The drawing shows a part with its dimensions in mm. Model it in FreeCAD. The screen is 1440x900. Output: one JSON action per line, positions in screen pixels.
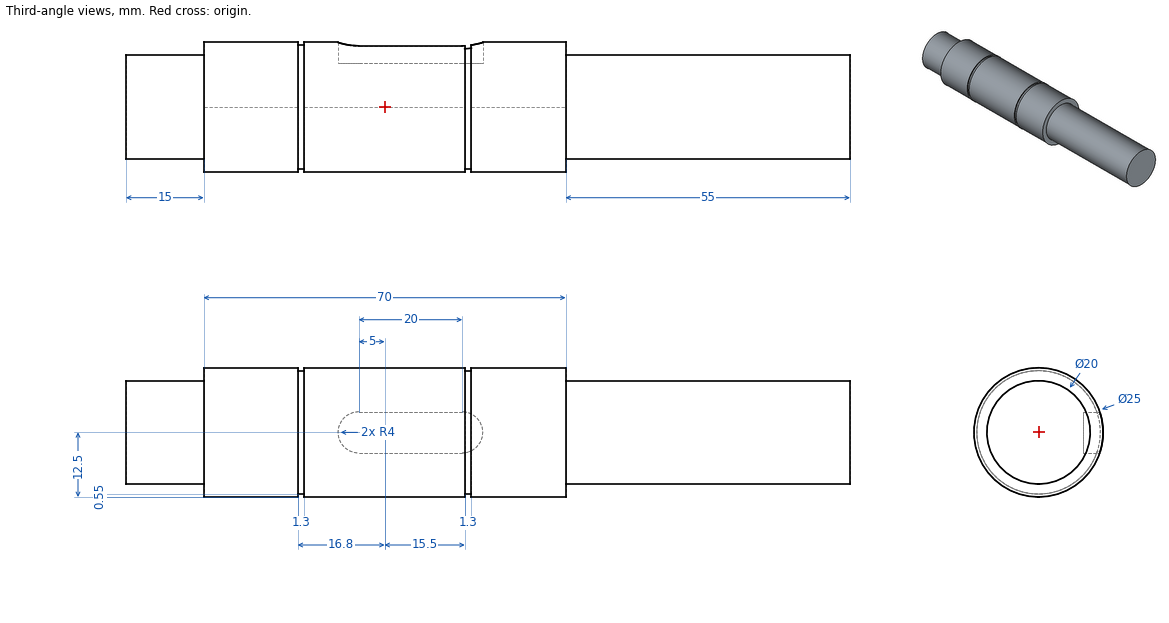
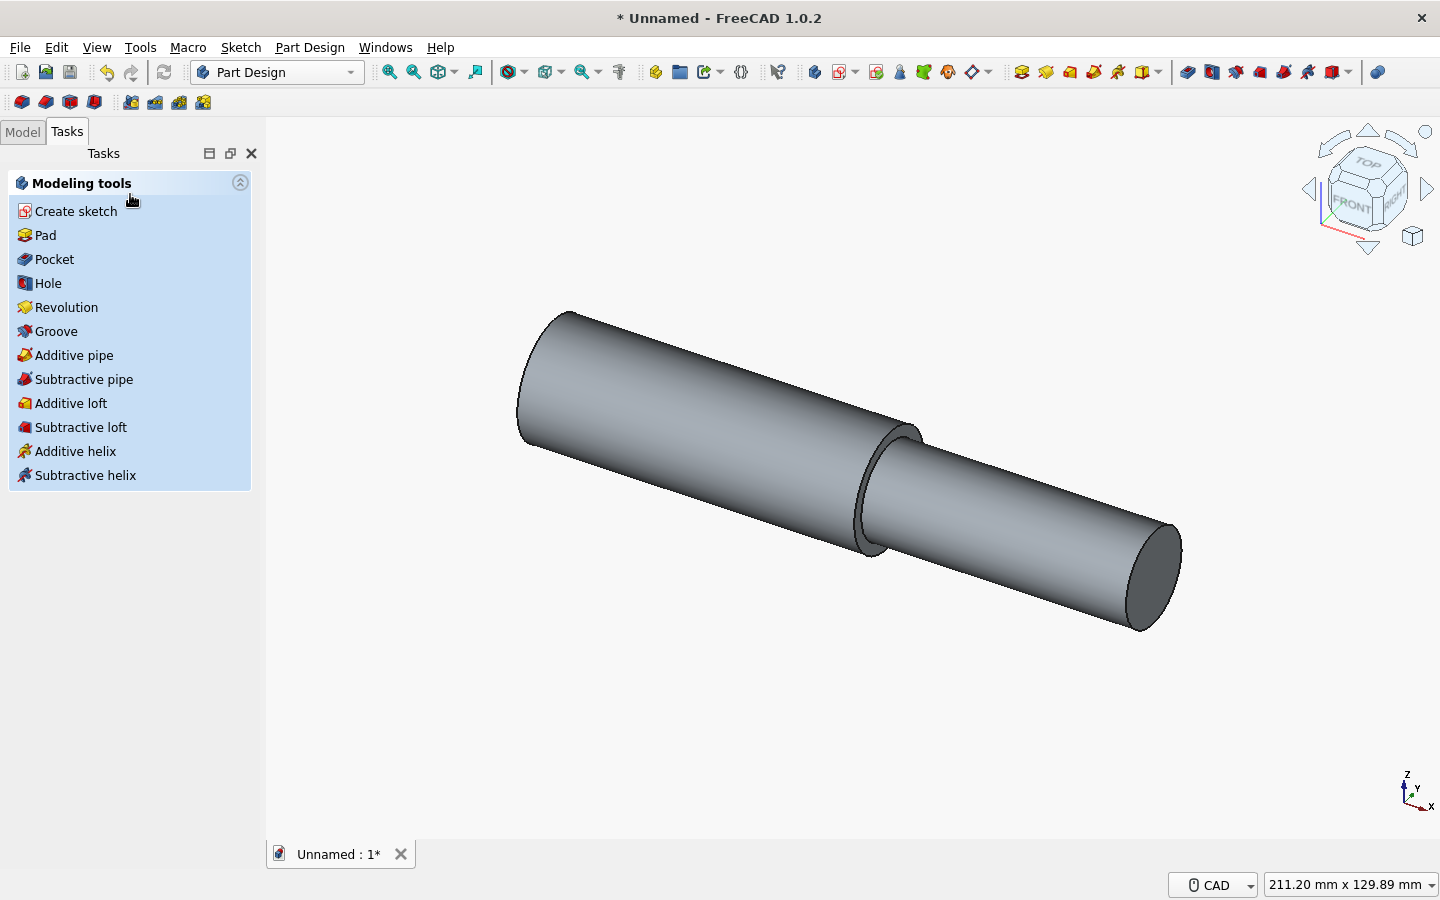
{"action": "left_click", "coordinate": [1236, 72]}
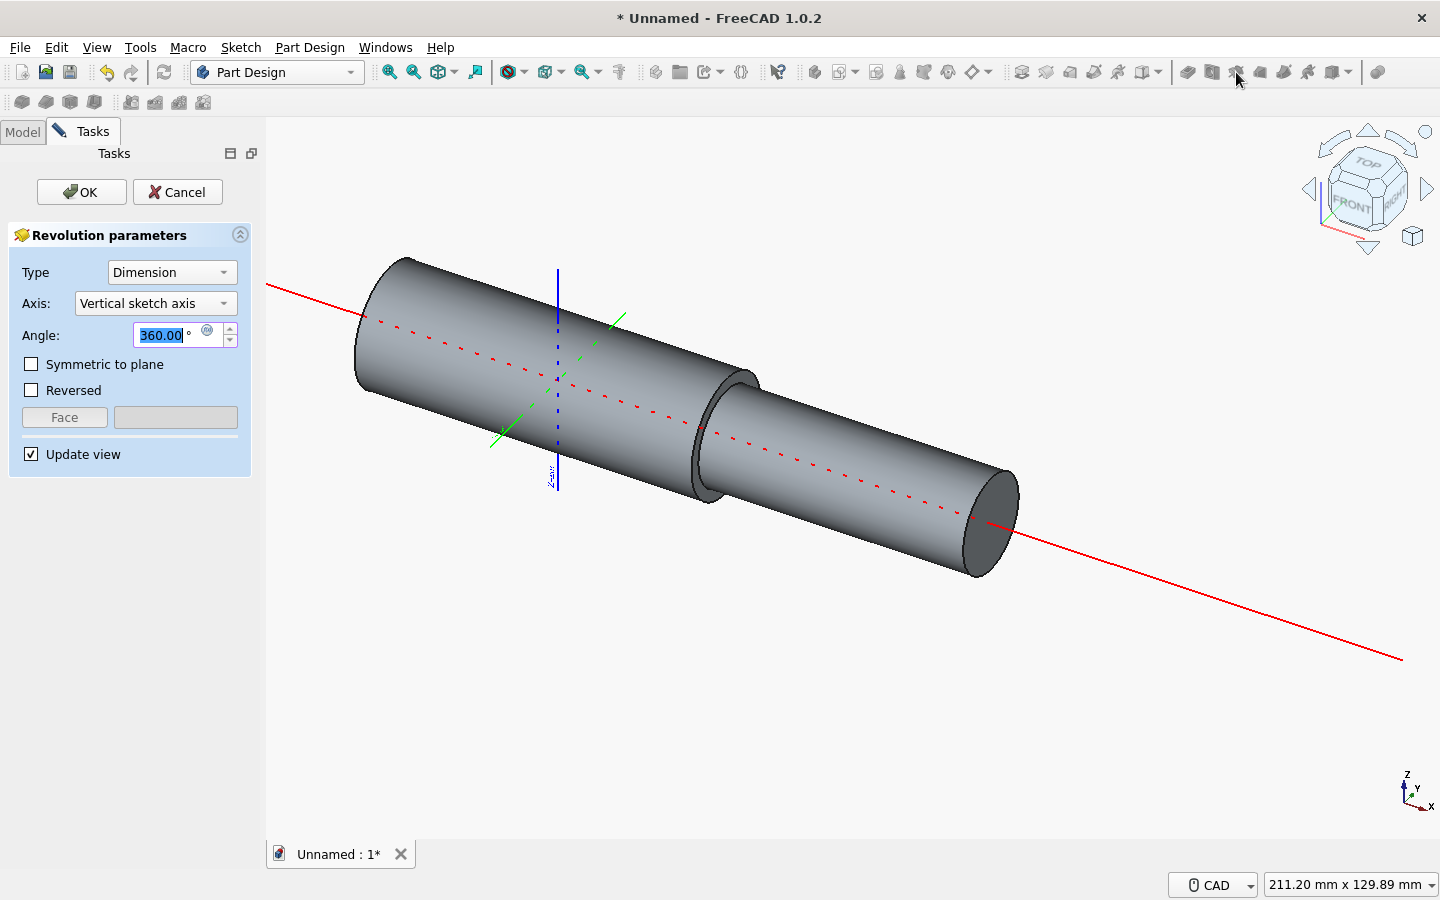
{"action": "left_click", "coordinate": [156, 304]}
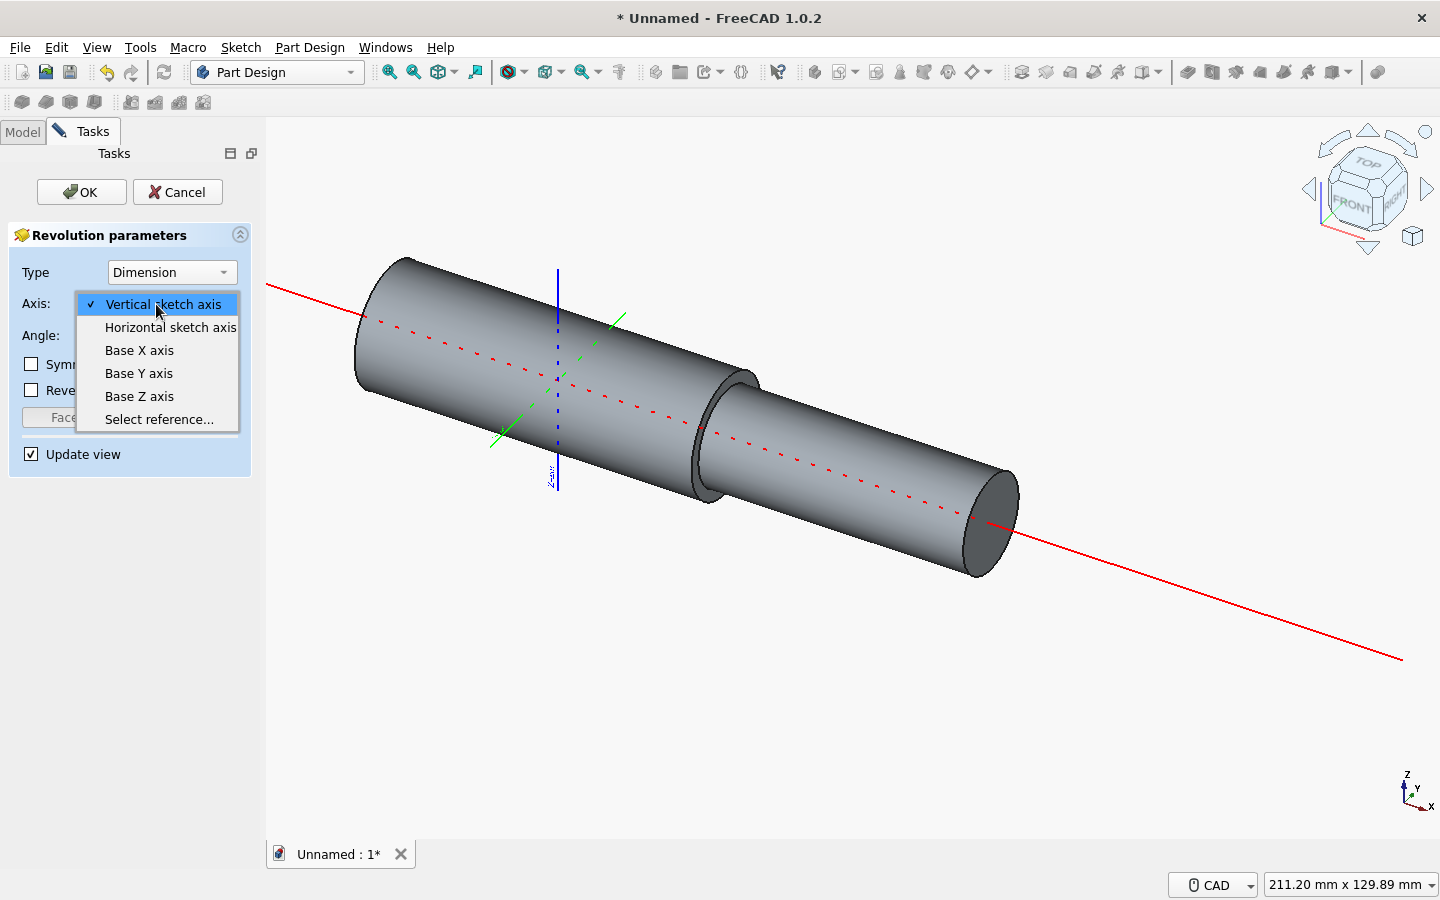
{"action": "left_click", "coordinate": [156, 328]}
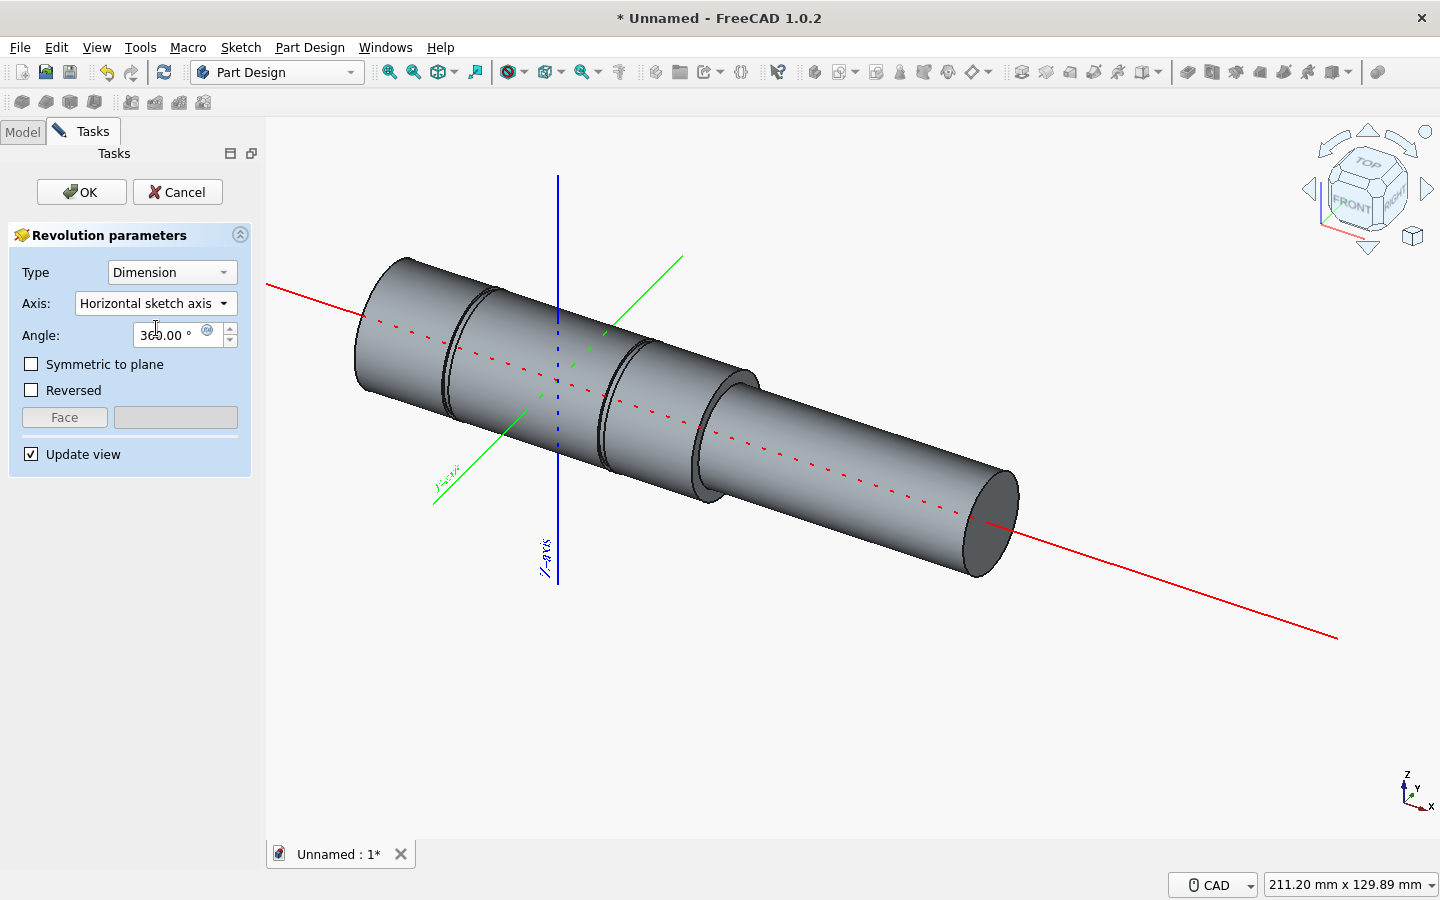
{"action": "left_click", "coordinate": [82, 192]}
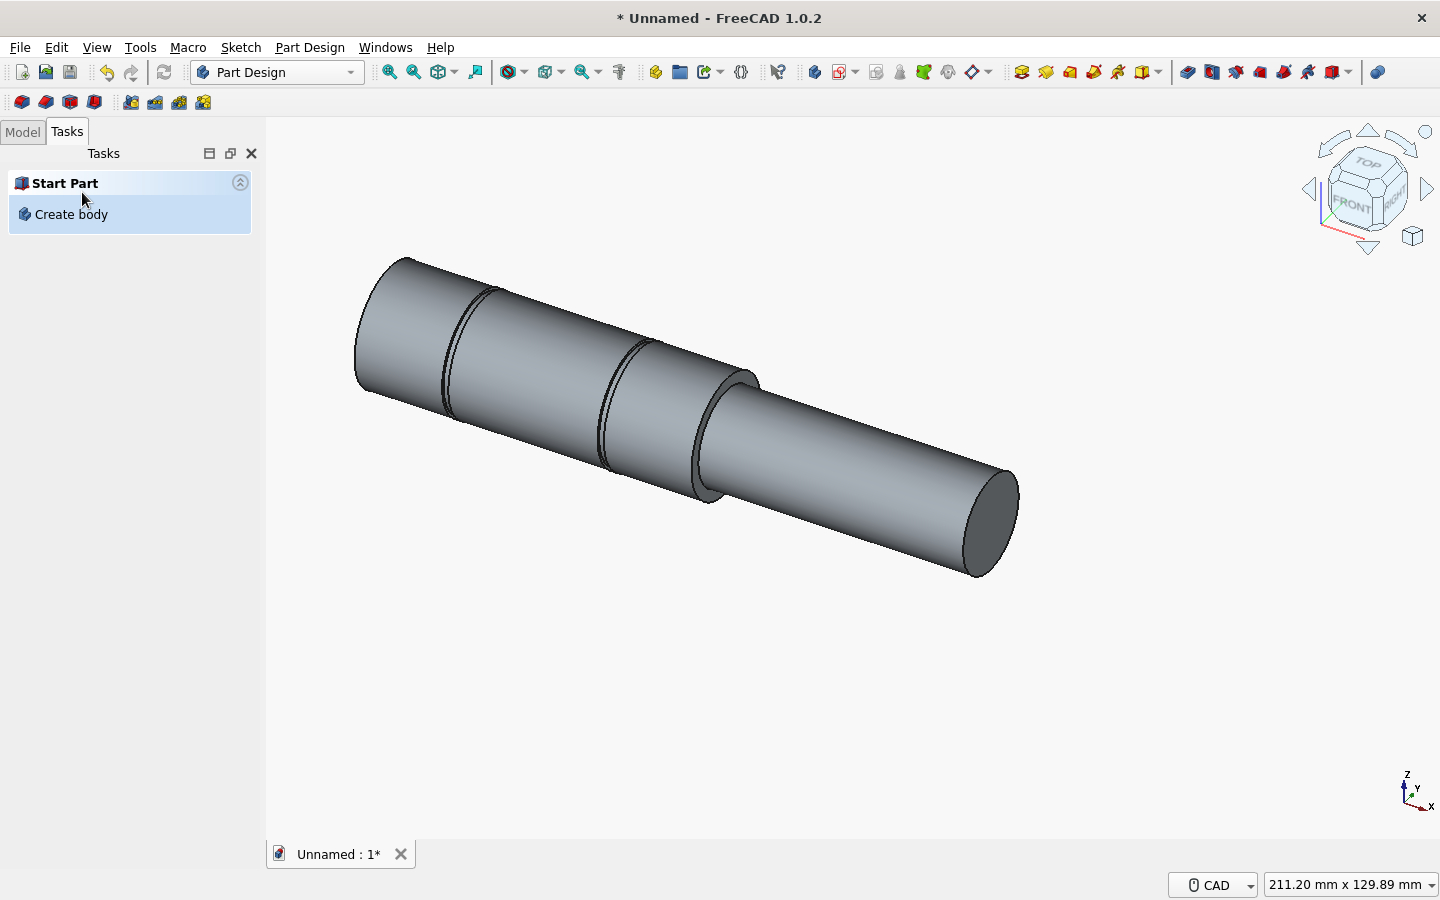
{"action": "left_click", "coordinate": [23, 131]}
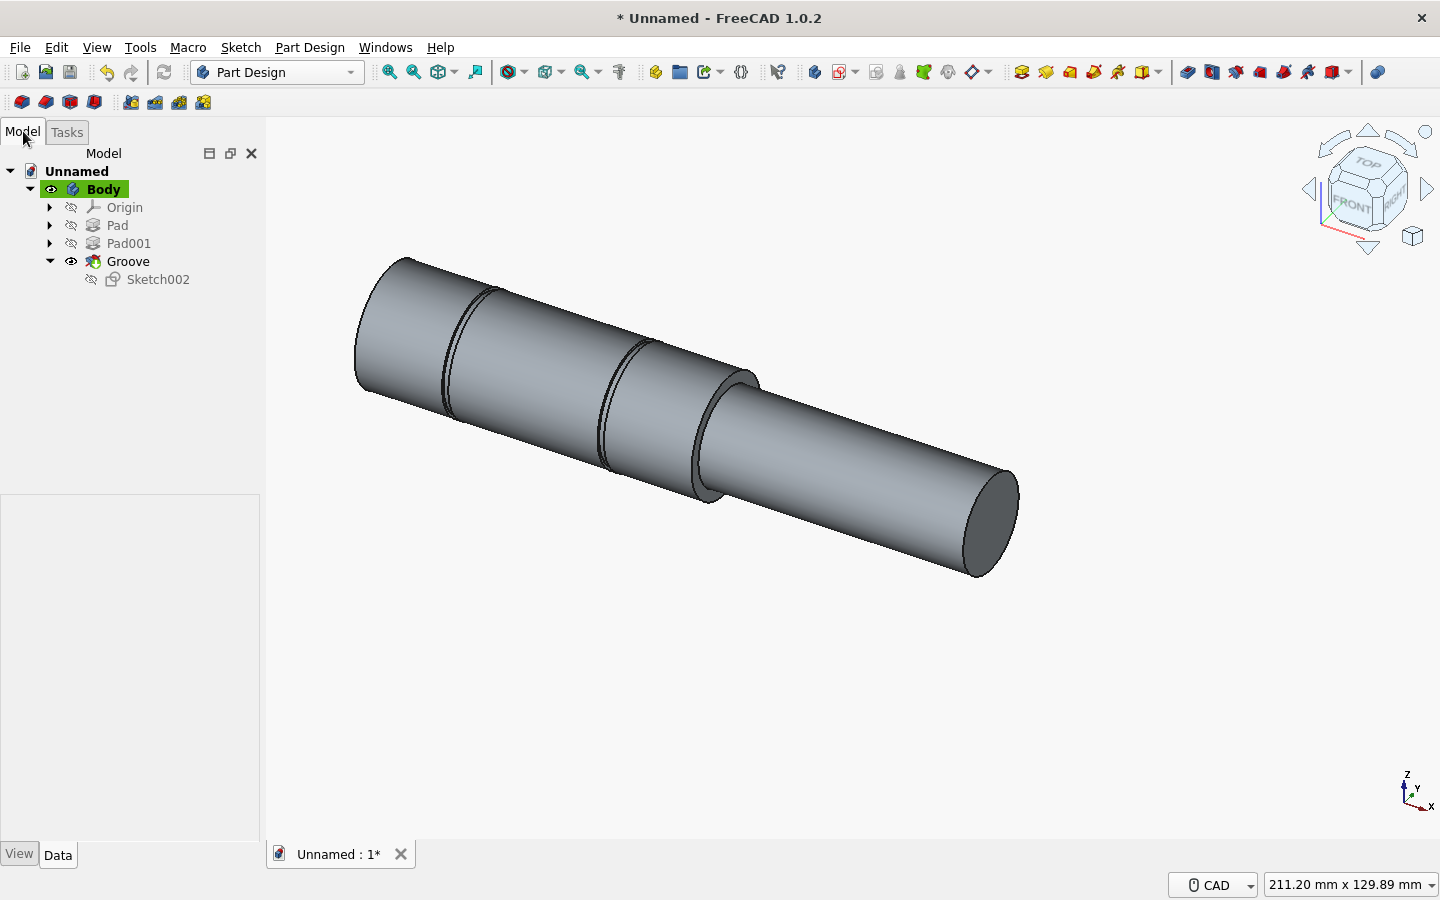
{"action": "left_click", "coordinate": [50, 207]}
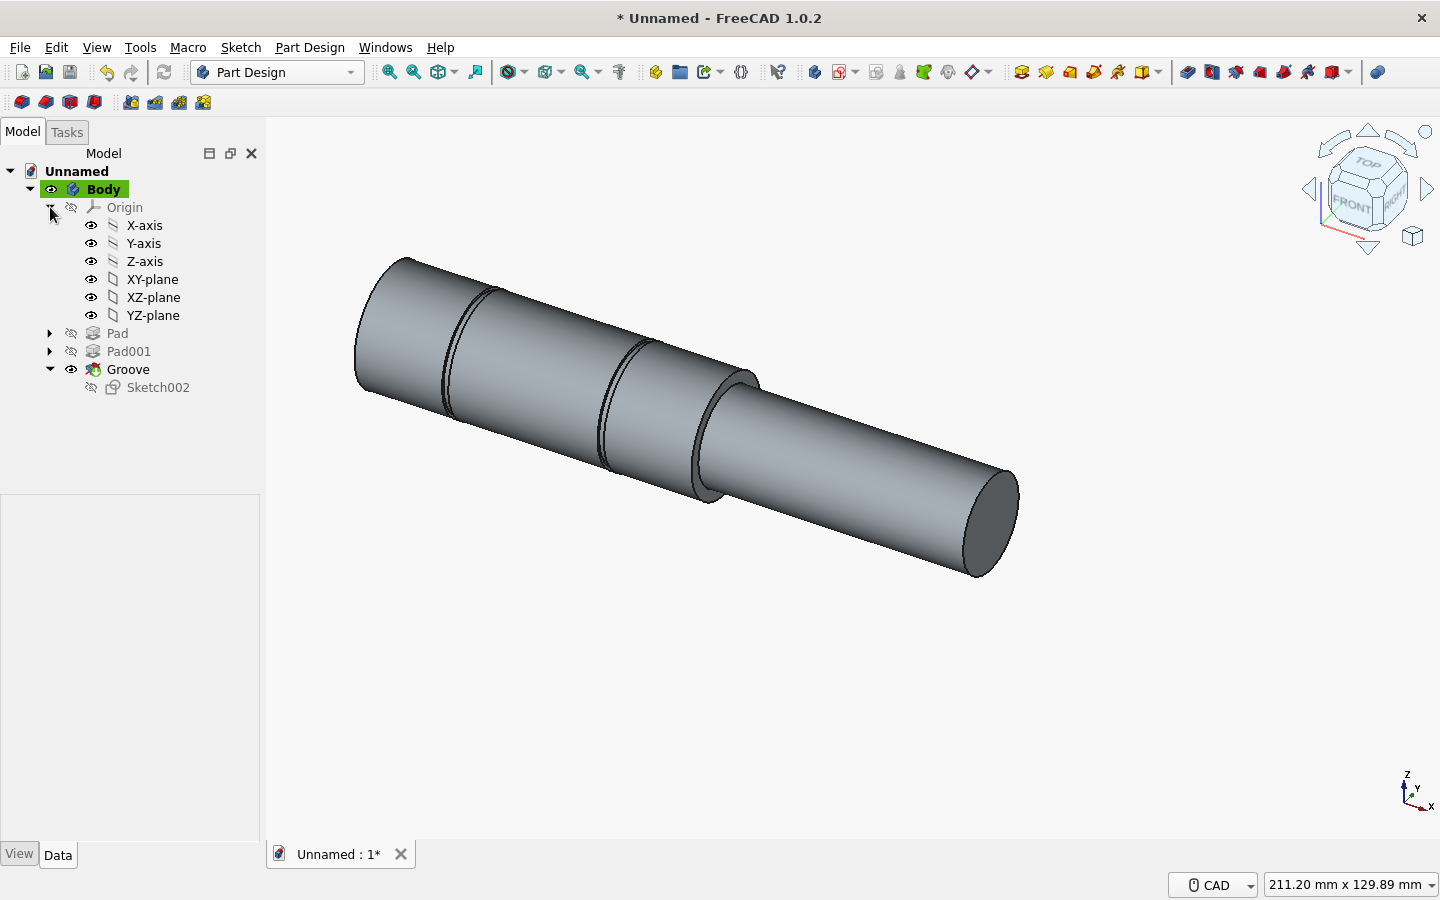
{"action": "left_click", "coordinate": [136, 297]}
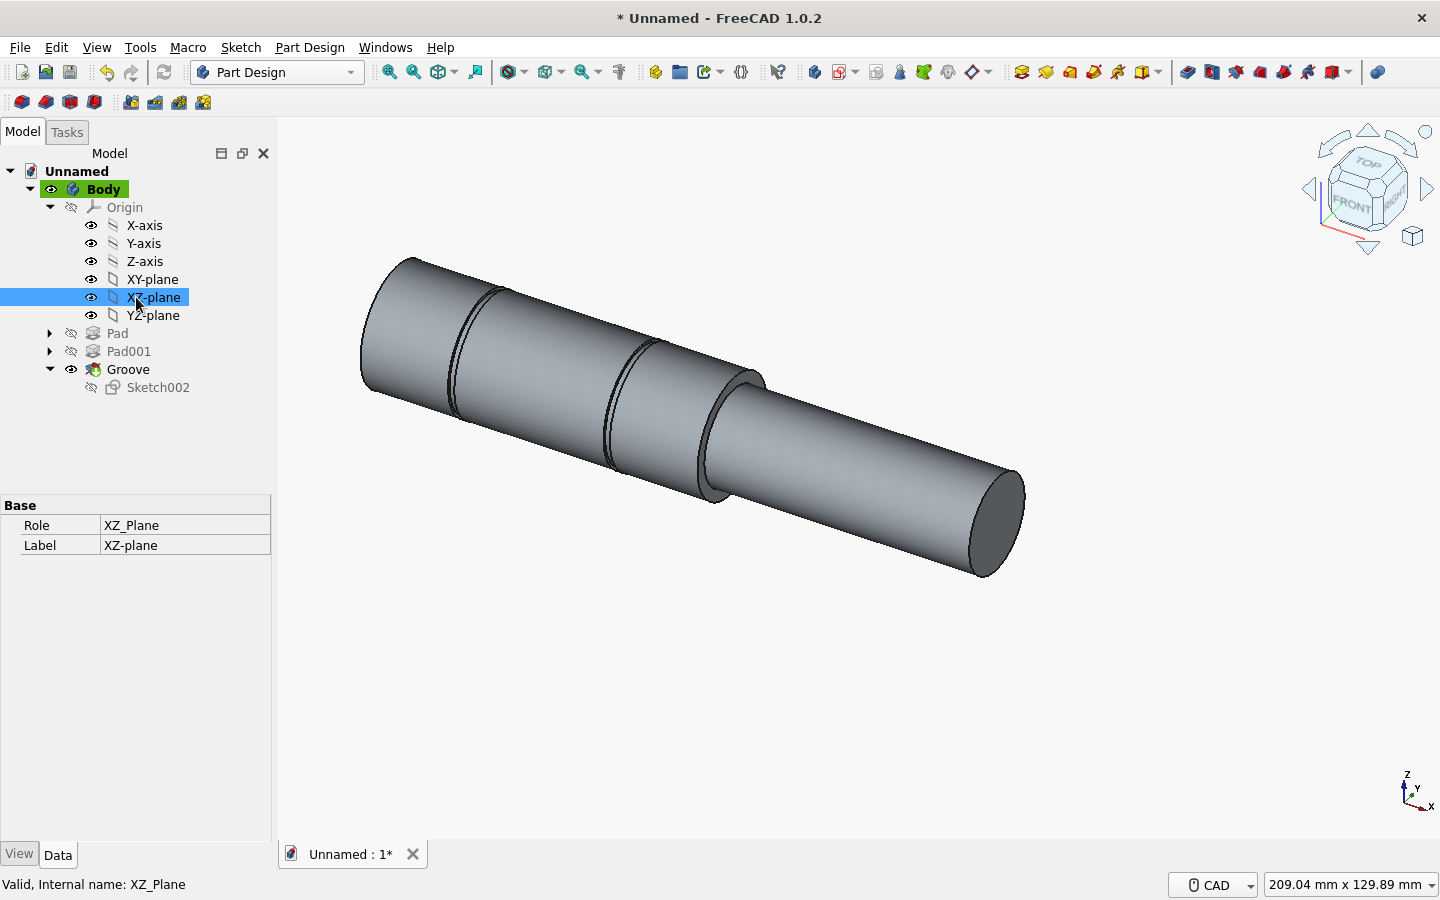
{"action": "left_click", "coordinate": [972, 72]}